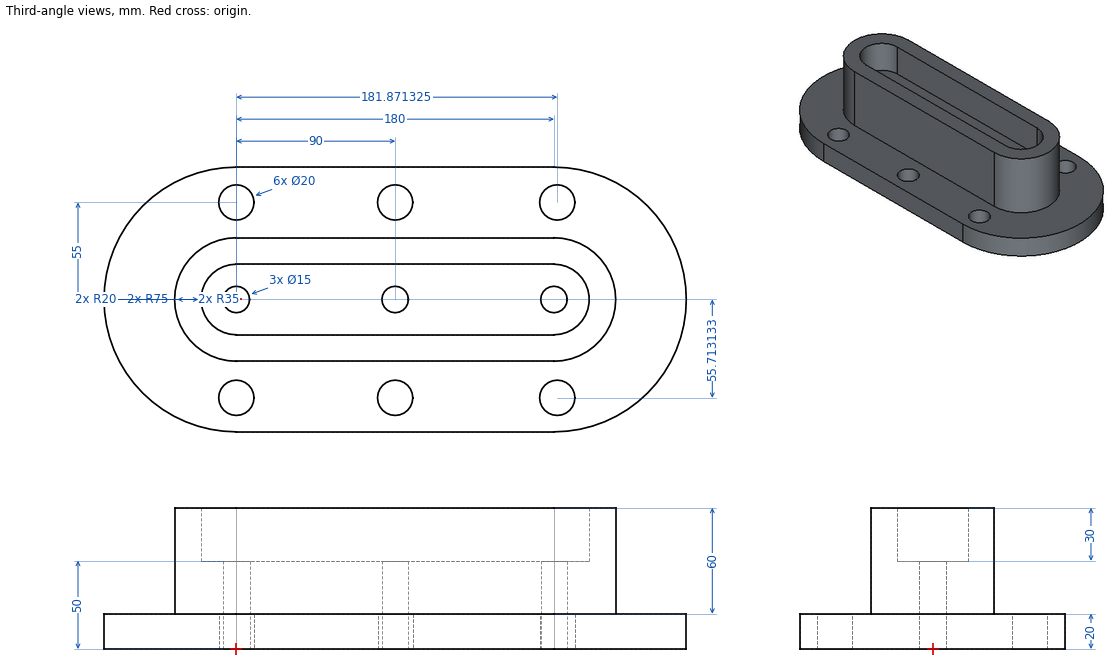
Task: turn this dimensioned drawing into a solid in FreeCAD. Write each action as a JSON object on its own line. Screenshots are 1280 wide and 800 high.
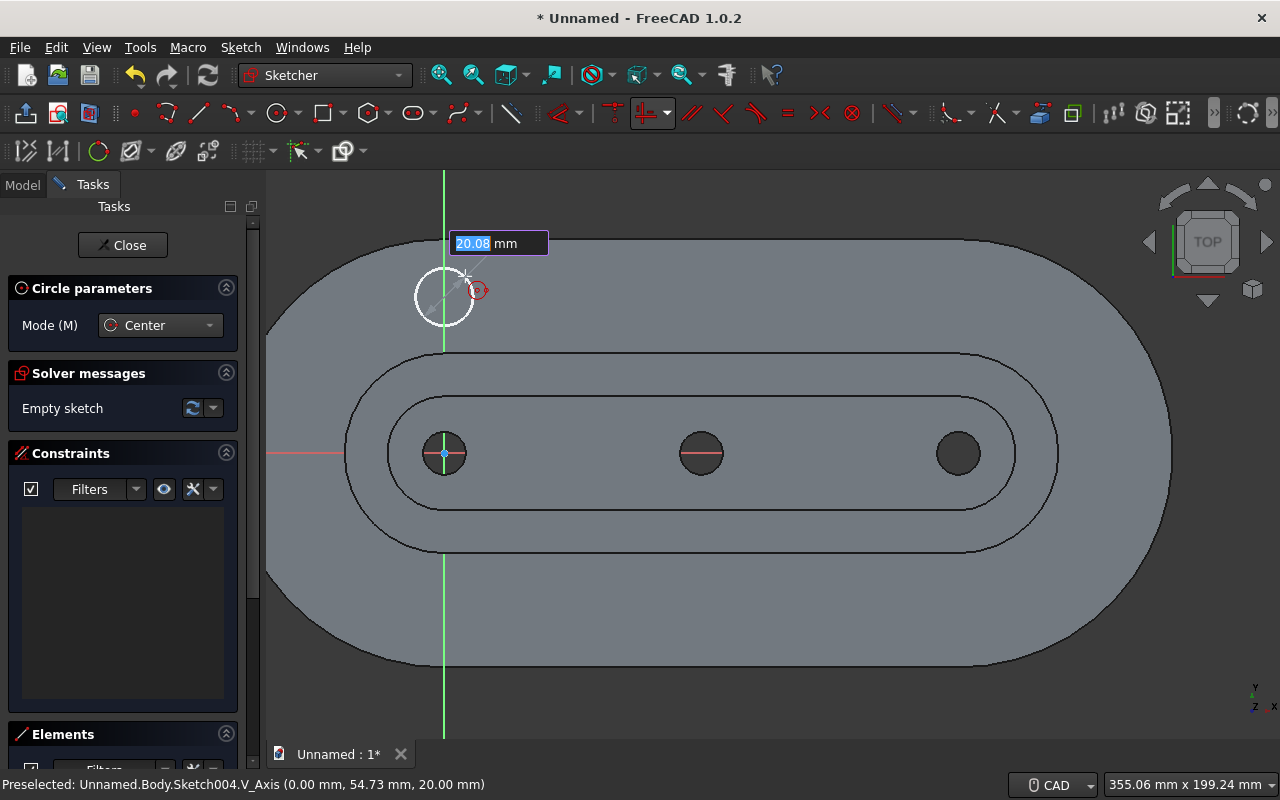
{"action": "type", "text": "20"}
{"action": "key", "text": "Return"}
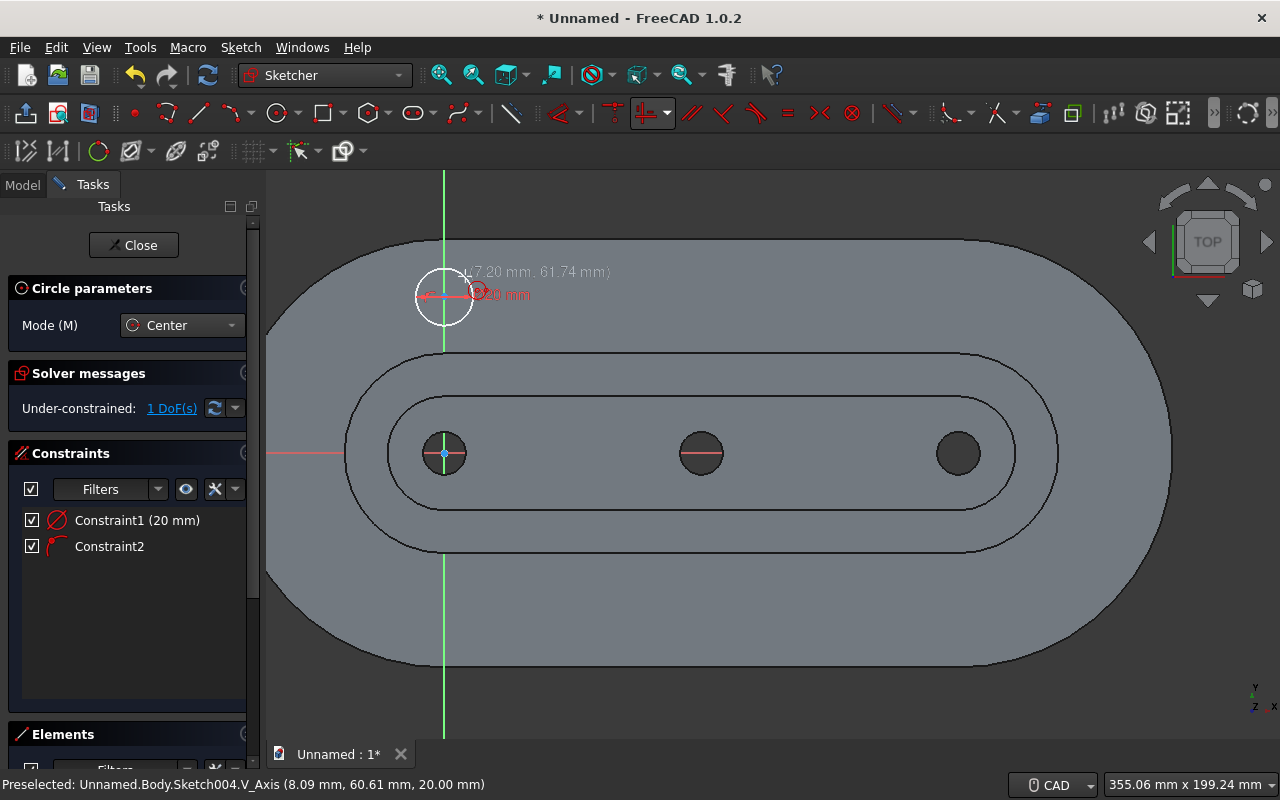
{"action": "left_click", "coordinate": [964, 296]}
{"action": "mouse_move", "coordinate": [984, 276]}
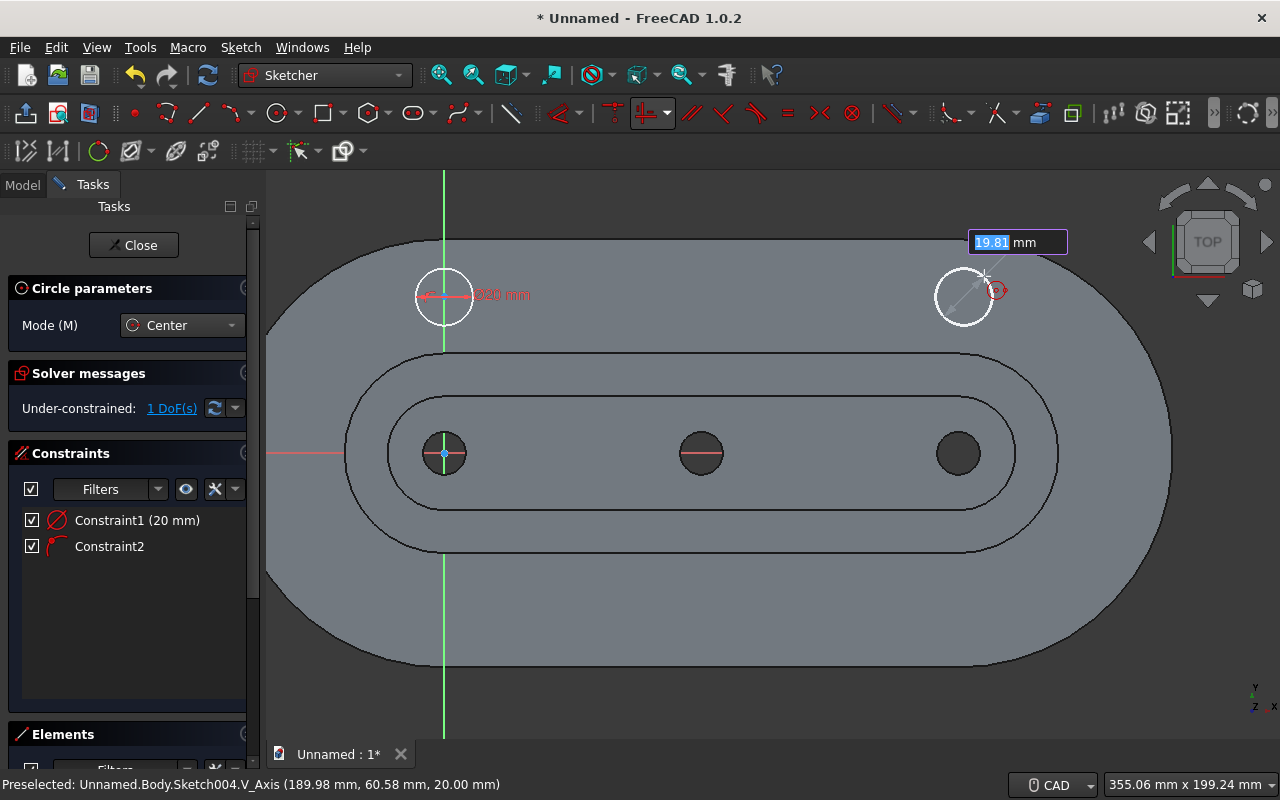
{"action": "type", "text": "20"}
{"action": "key", "text": "Return"}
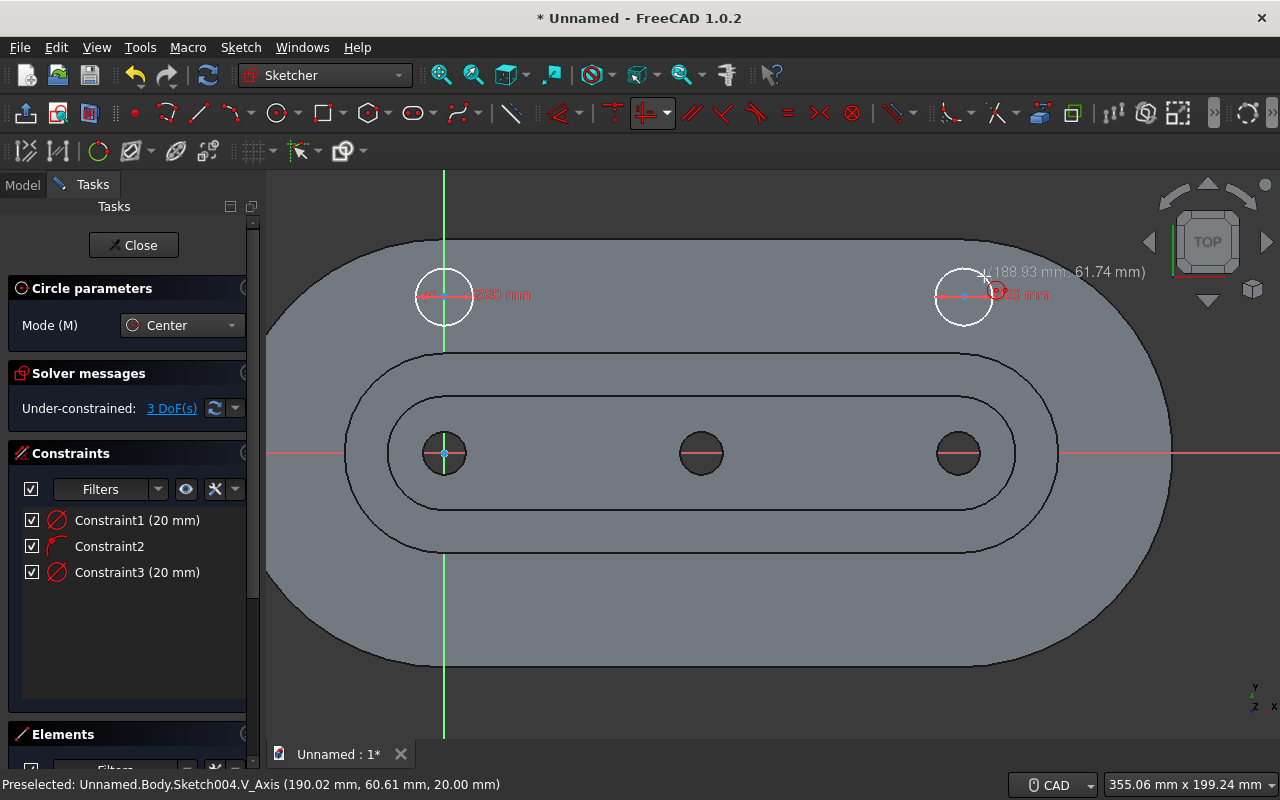
{"action": "left_click", "coordinate": [964, 612]}
{"action": "mouse_move", "coordinate": [984, 592]}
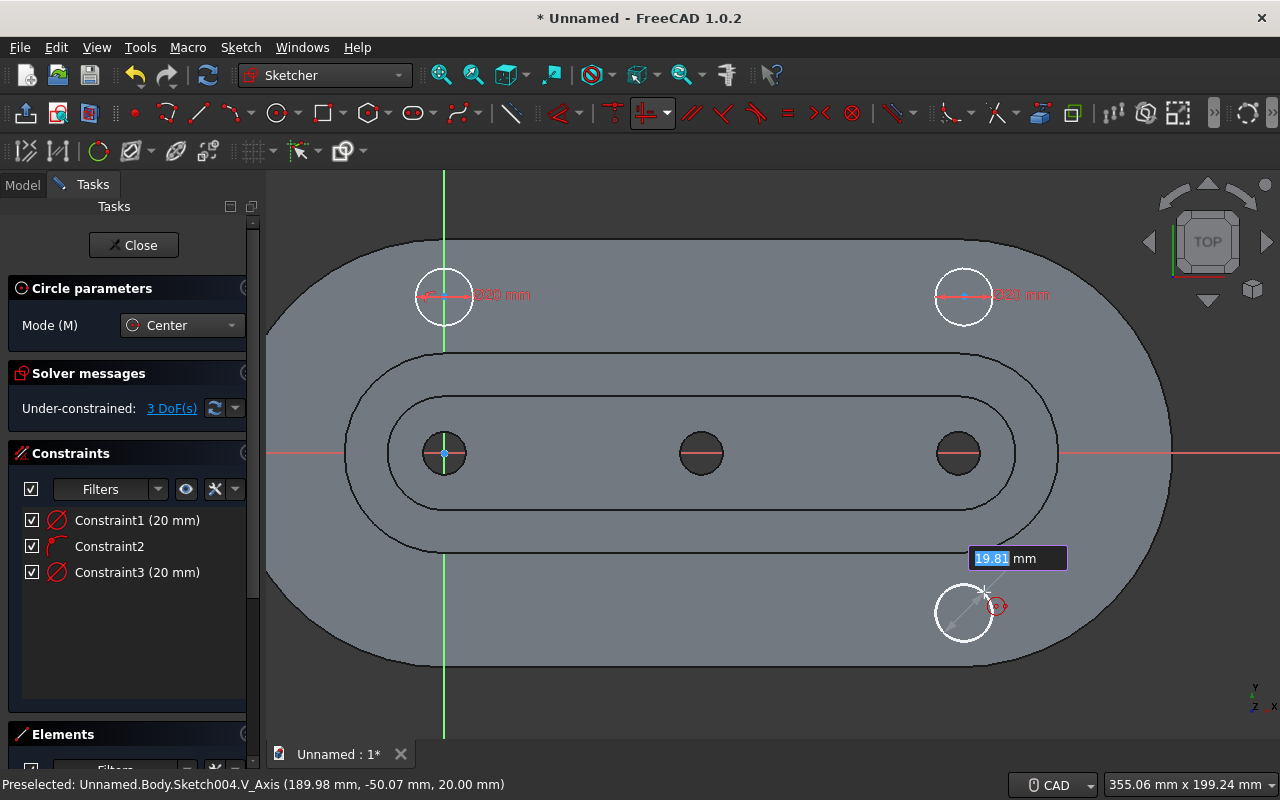
{"action": "type", "text": "20"}
{"action": "key", "text": "Return"}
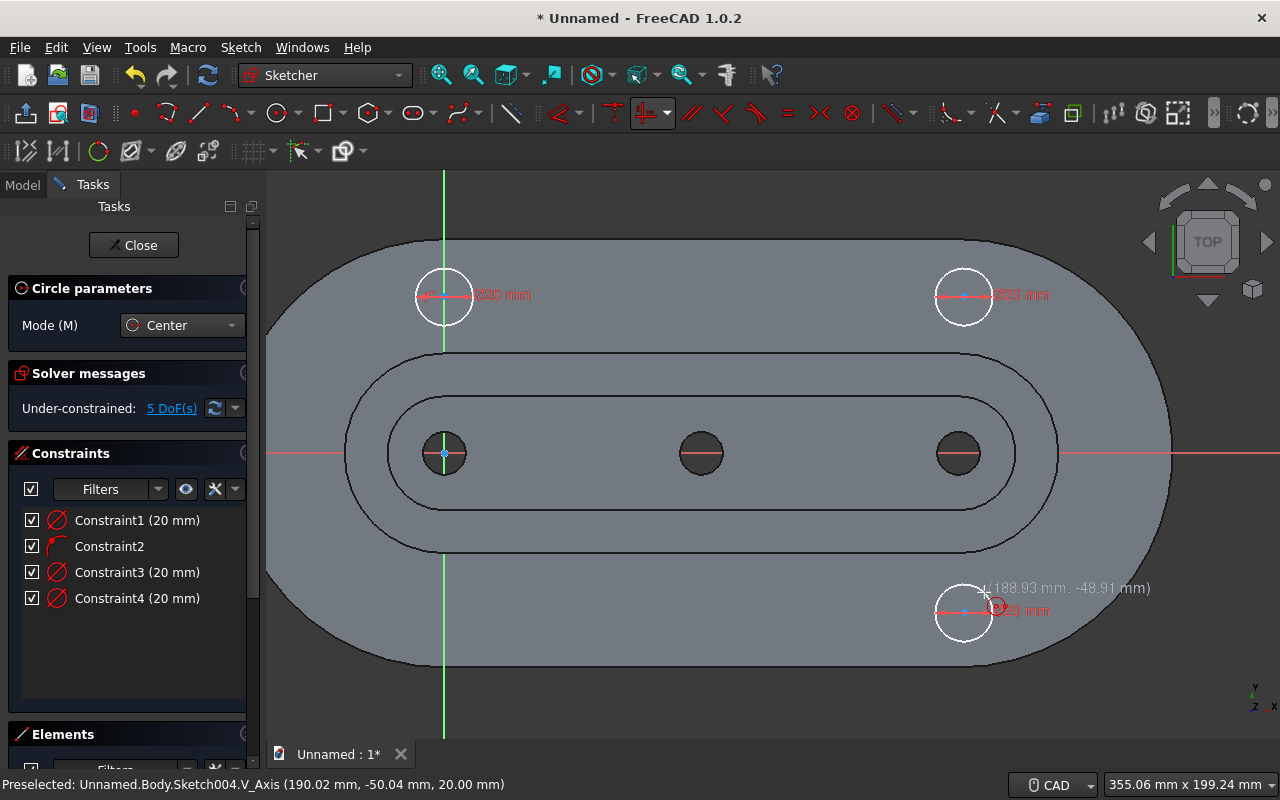
{"action": "left_click", "coordinate": [444, 612]}
{"action": "mouse_move", "coordinate": [465, 592]}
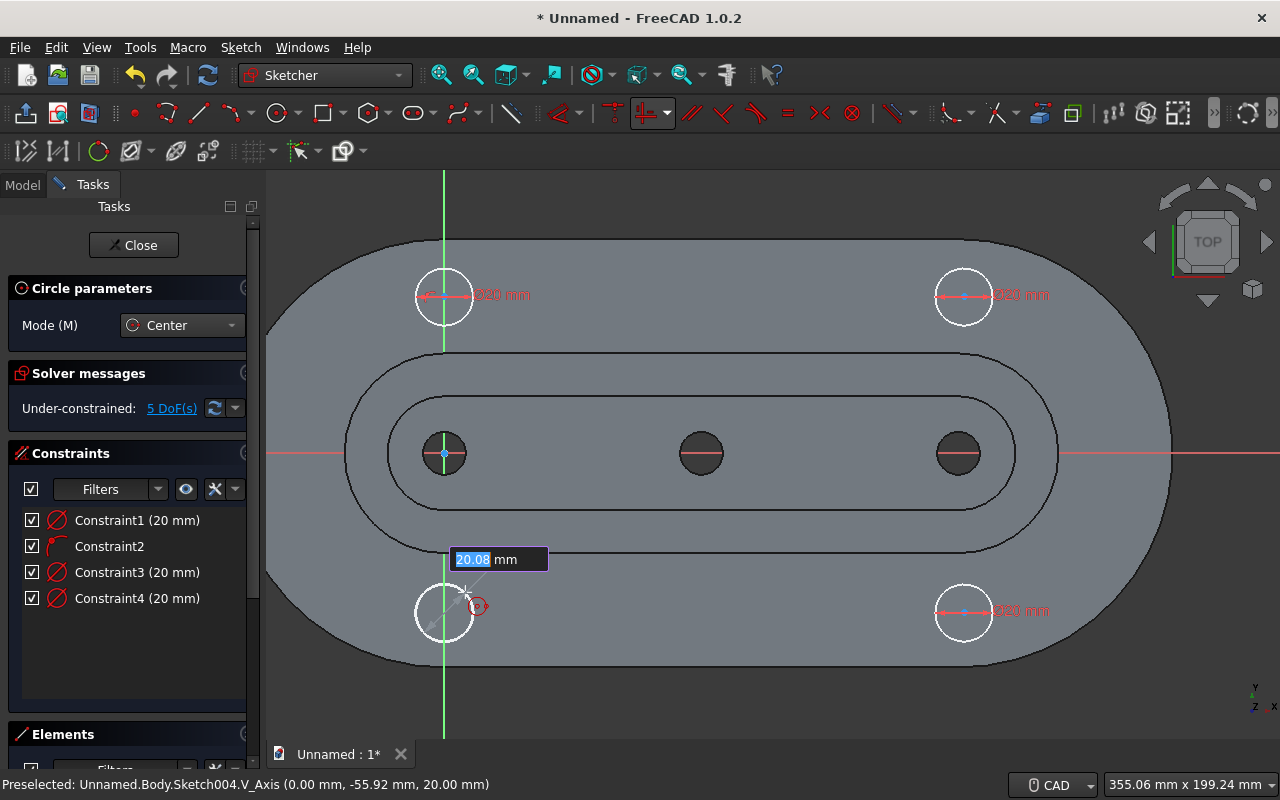
{"action": "type", "text": "20"}
{"action": "key", "text": "Return"}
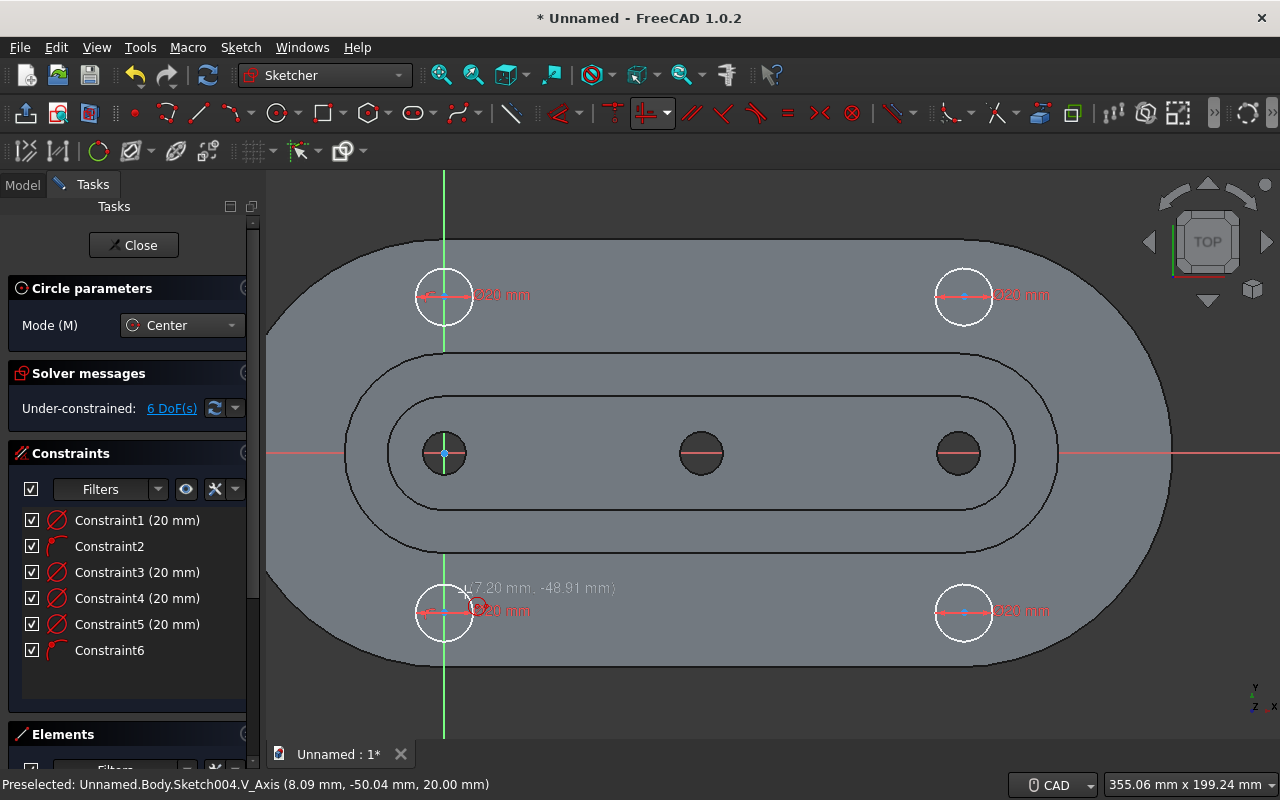
{"action": "left_click", "coordinate": [701, 296]}
{"action": "mouse_move", "coordinate": [722, 276]}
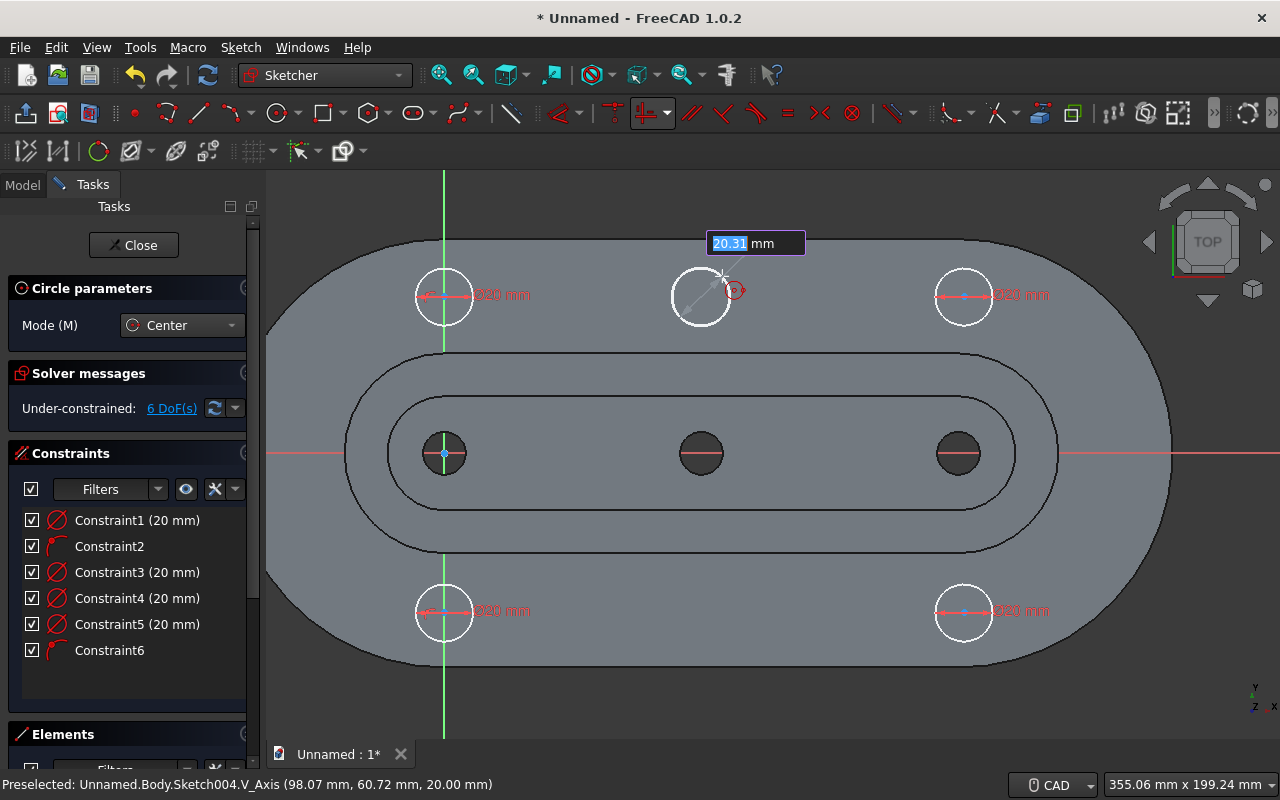
{"action": "type", "text": "20"}
{"action": "key", "text": "Return"}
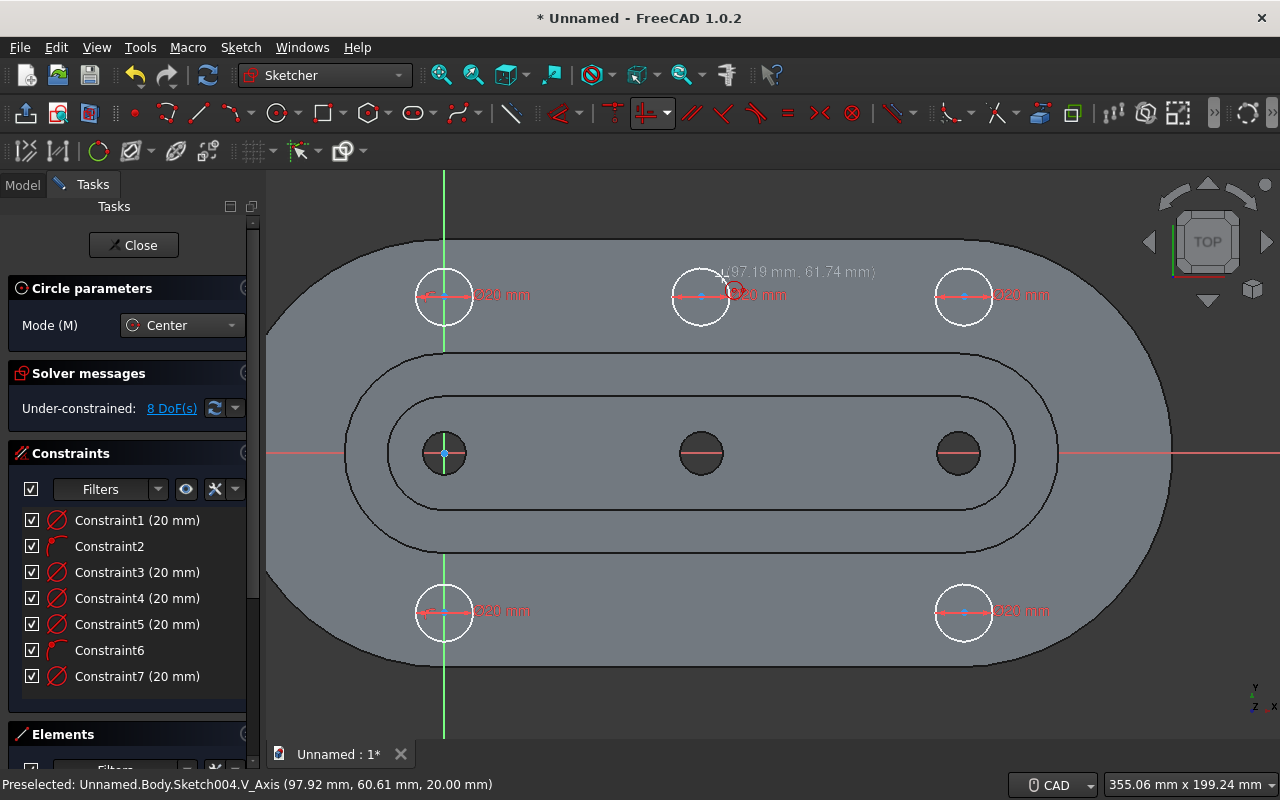
{"action": "left_click", "coordinate": [701, 612]}
{"action": "mouse_move", "coordinate": [722, 592]}